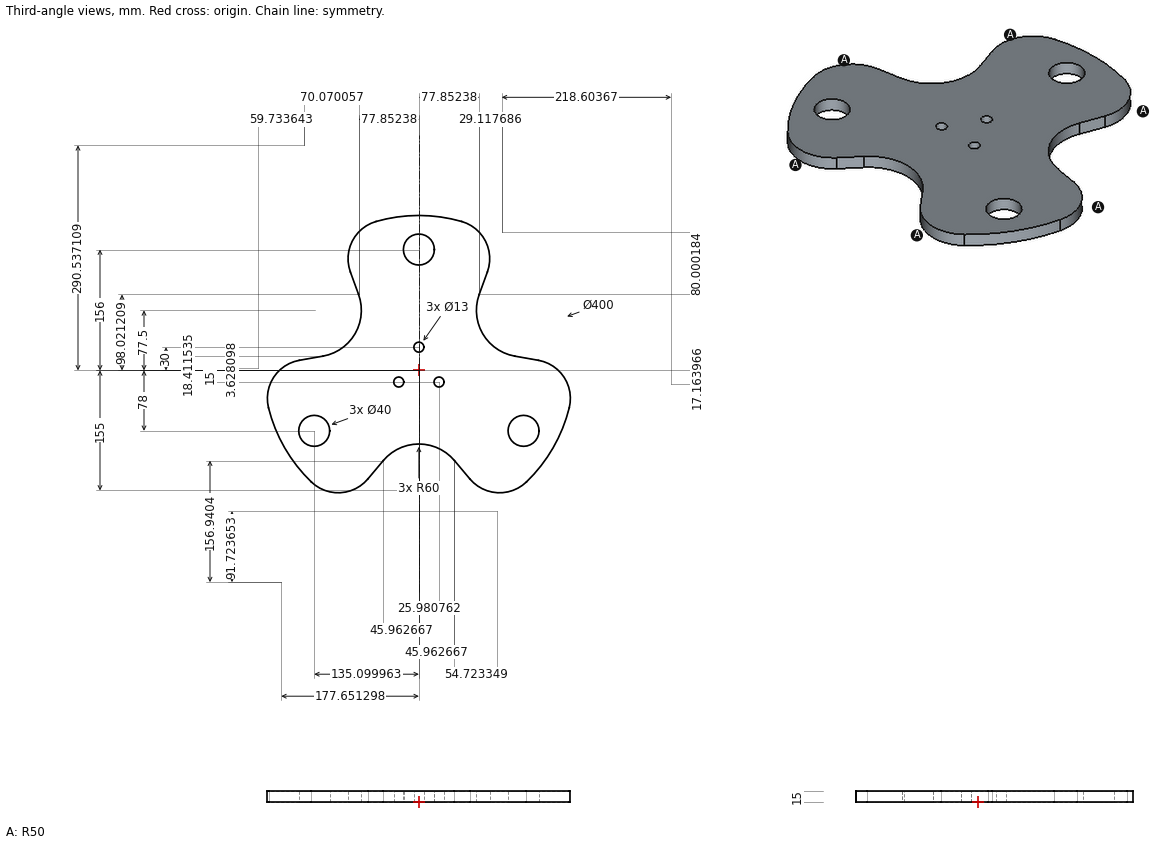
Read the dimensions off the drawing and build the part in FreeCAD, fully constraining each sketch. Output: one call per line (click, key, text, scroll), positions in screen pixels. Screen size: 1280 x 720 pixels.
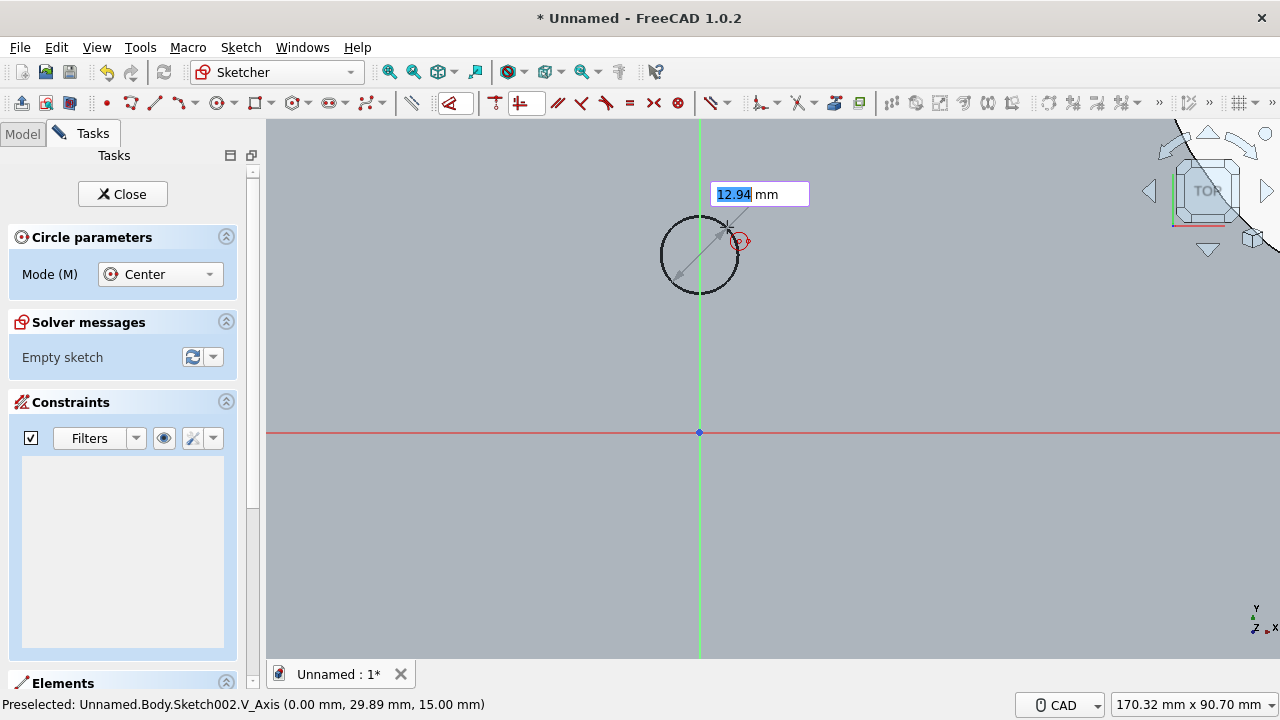
text(13)
key(Return)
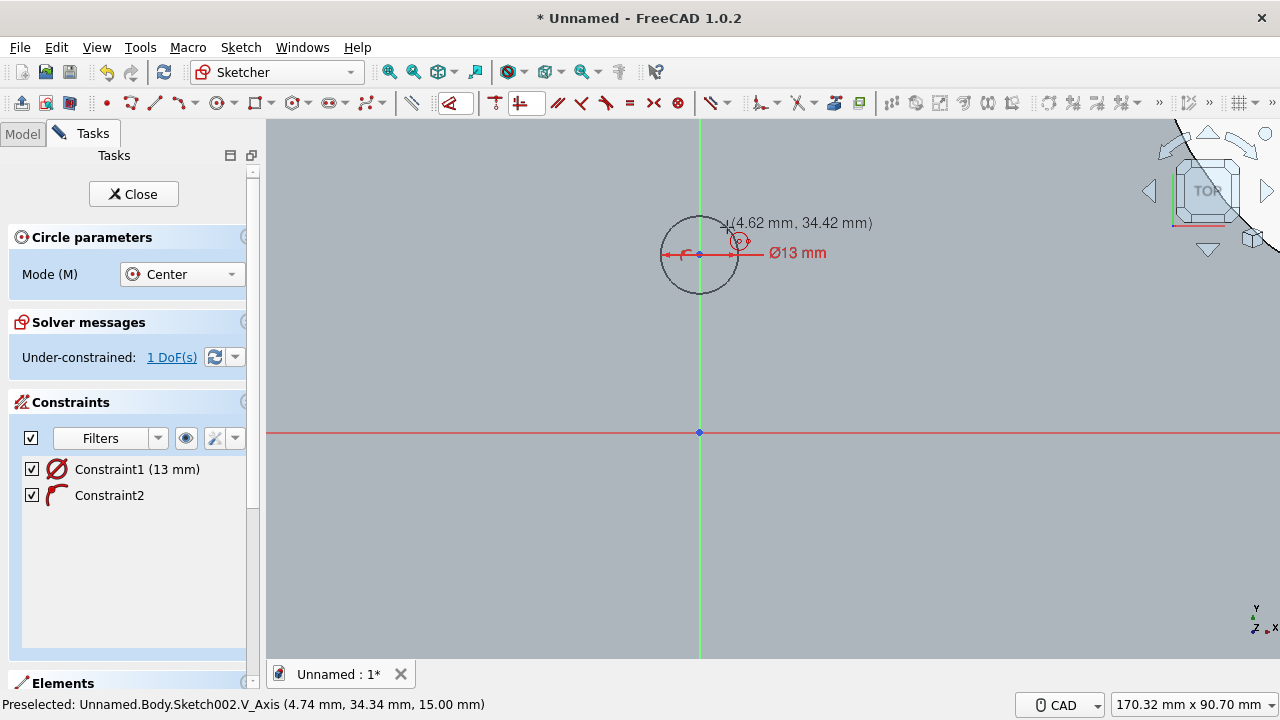
click(854, 522)
move(882, 495)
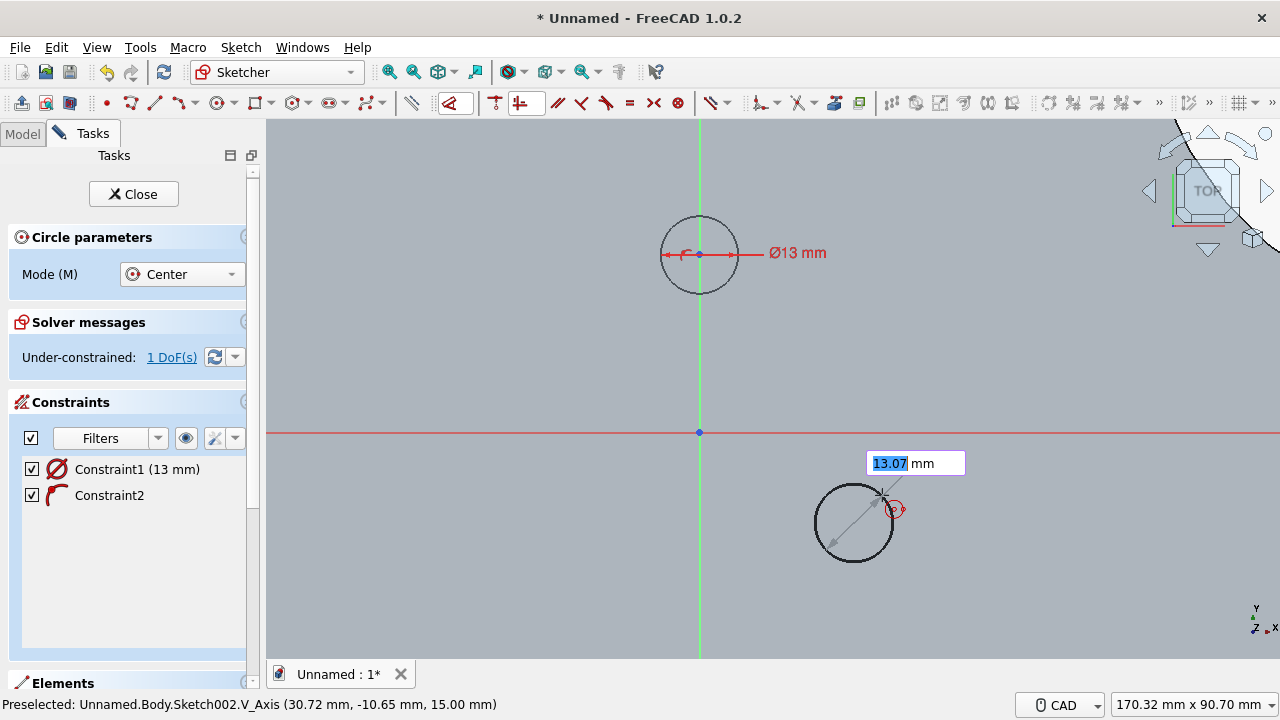
text(13)
key(Return)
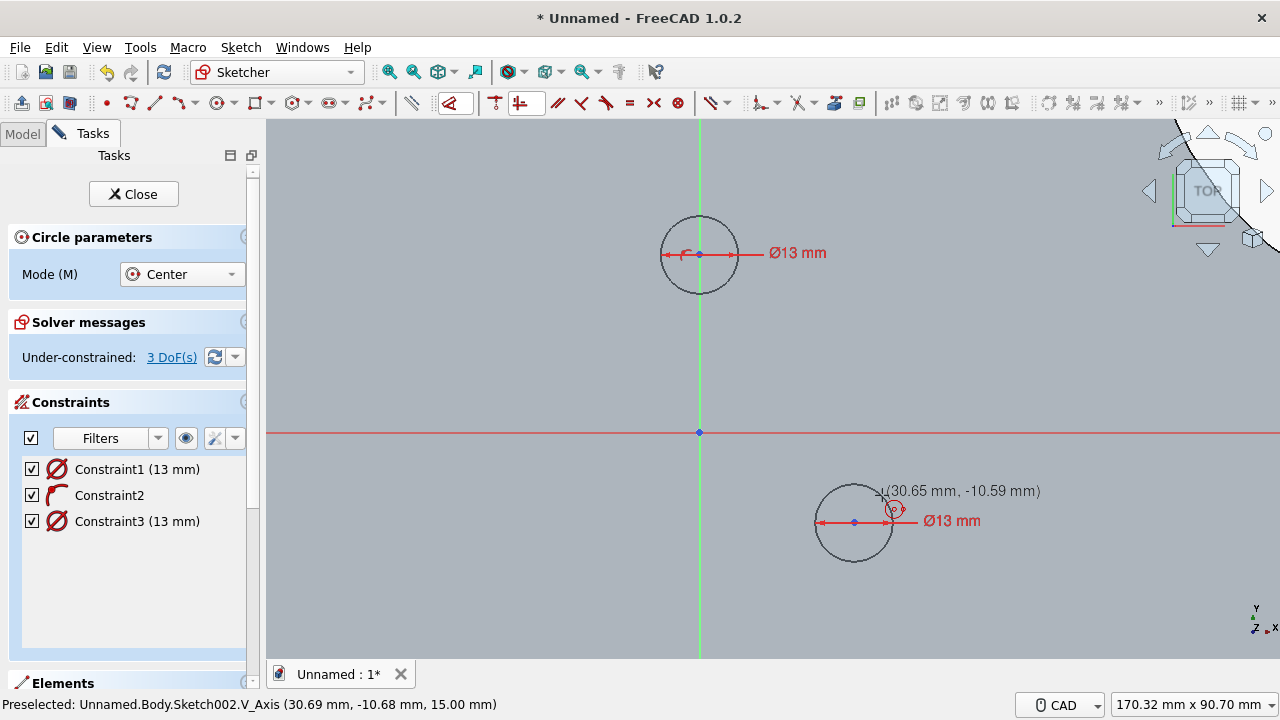
click(545, 522)
move(572, 495)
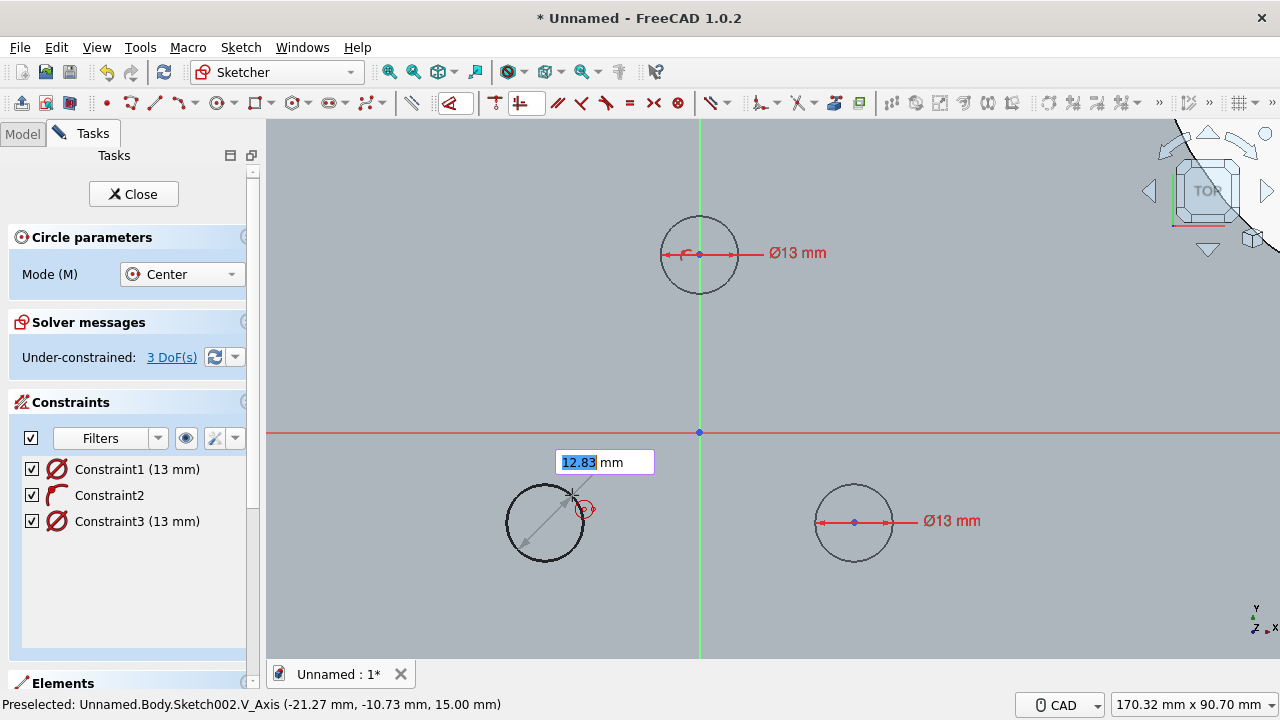
text(13)
key(Return)
key(Escape)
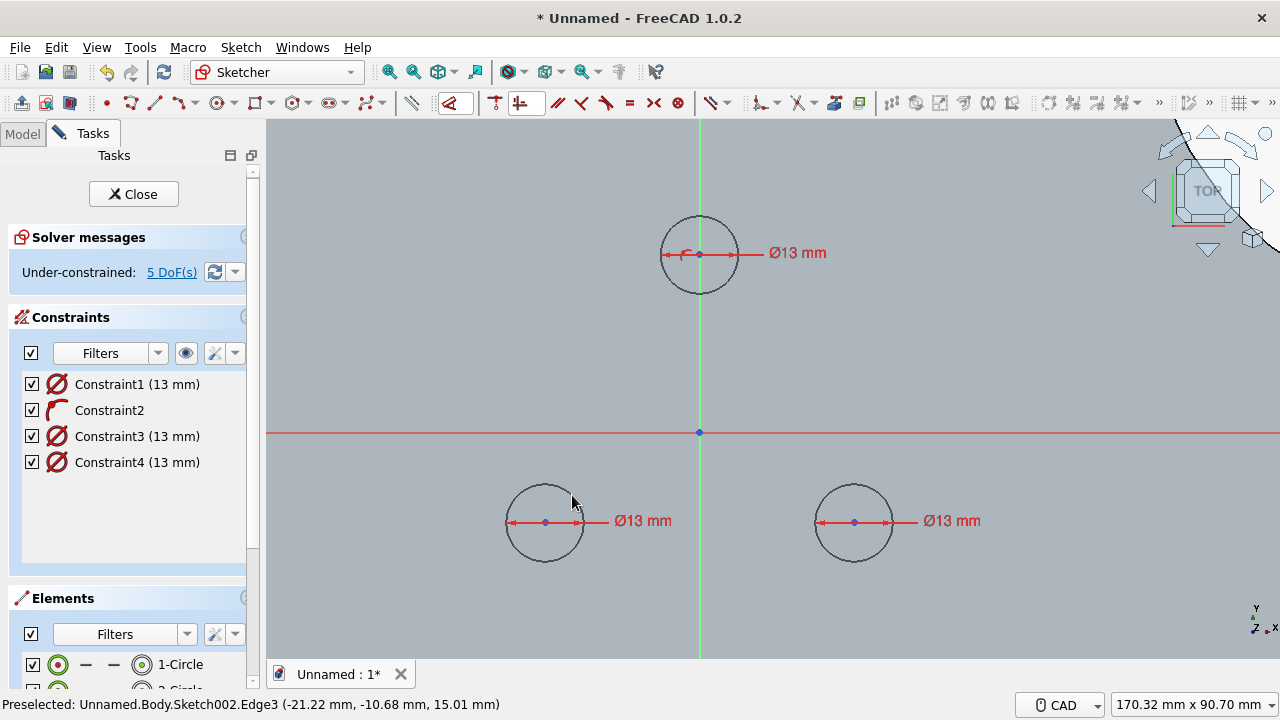
click(854, 523)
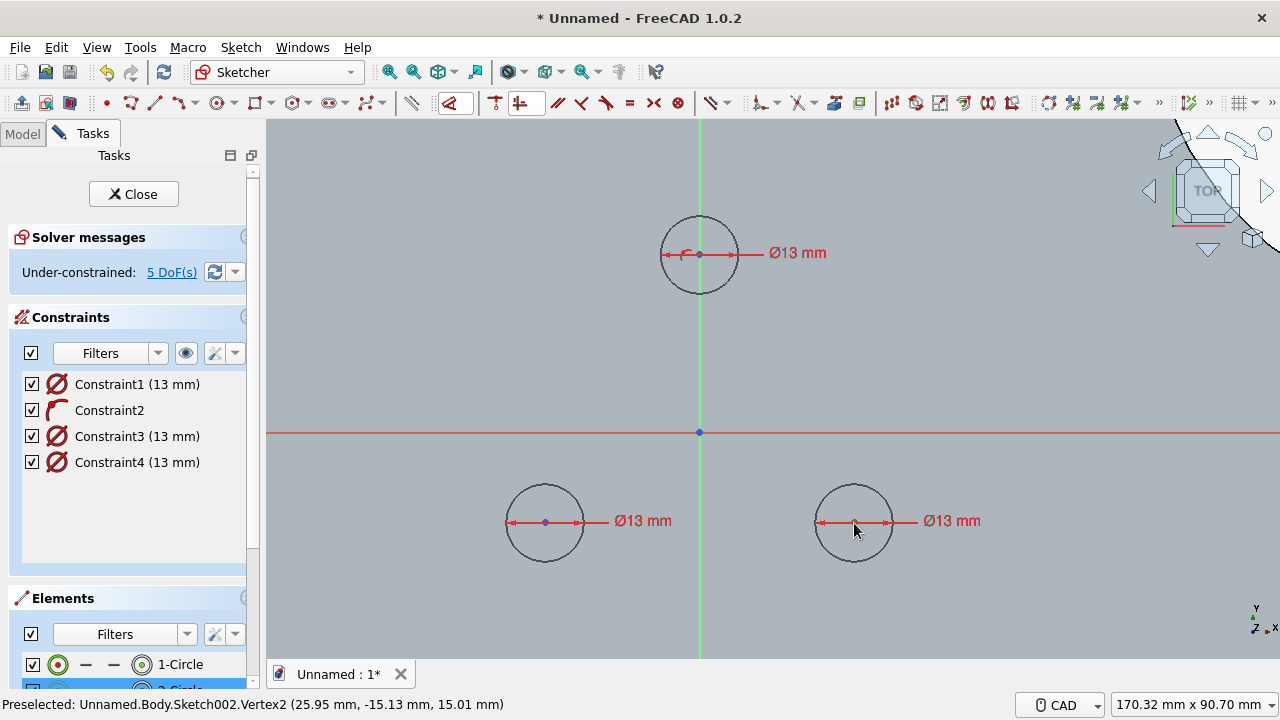
click(545, 523)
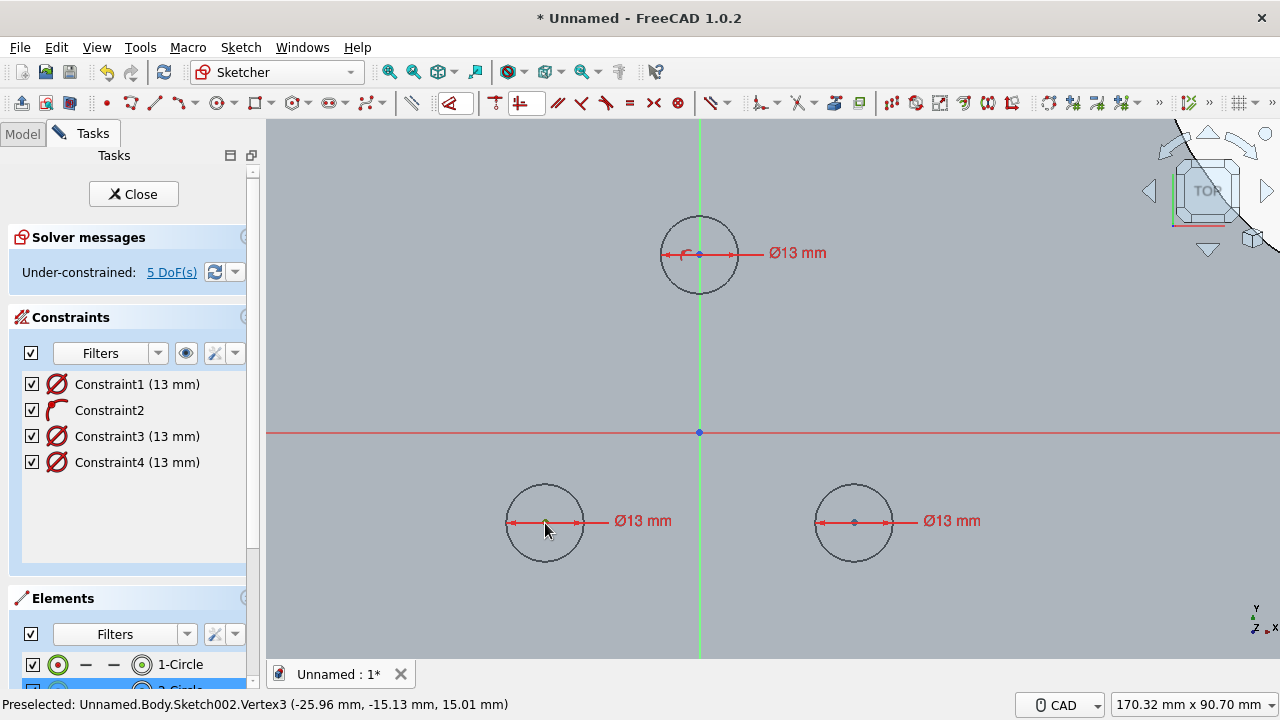
click(700, 596)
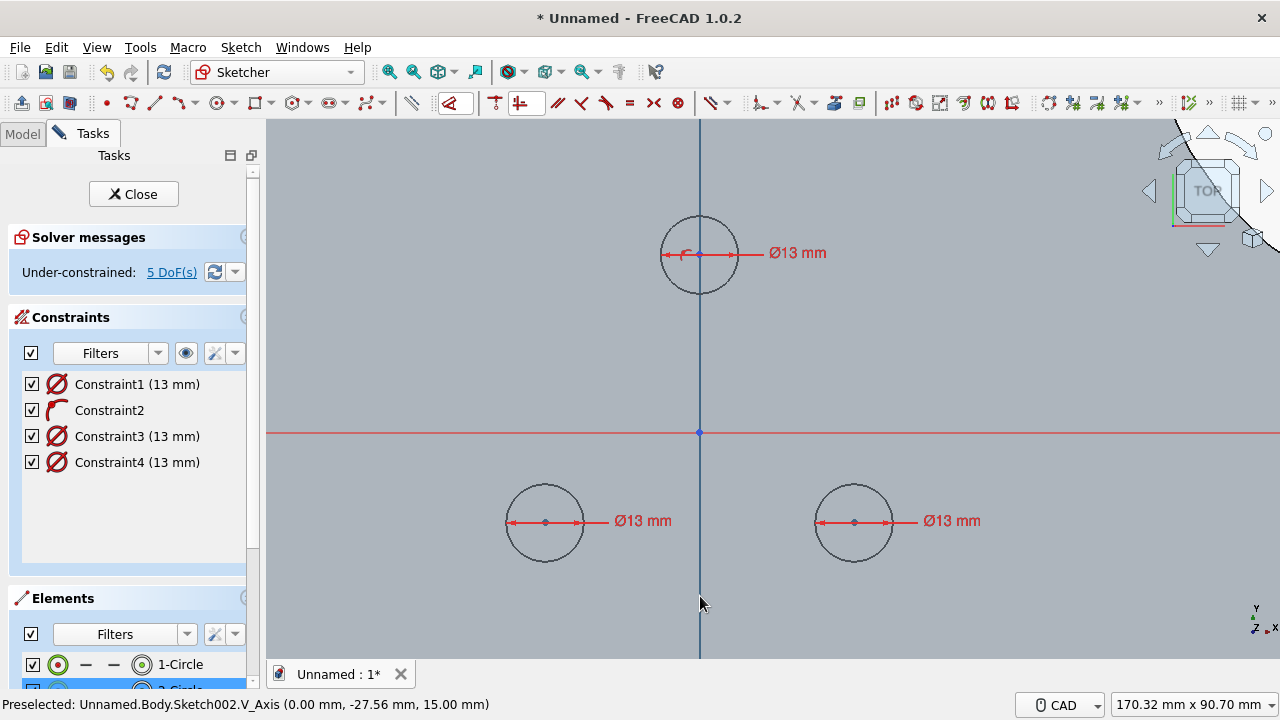
click(654, 104)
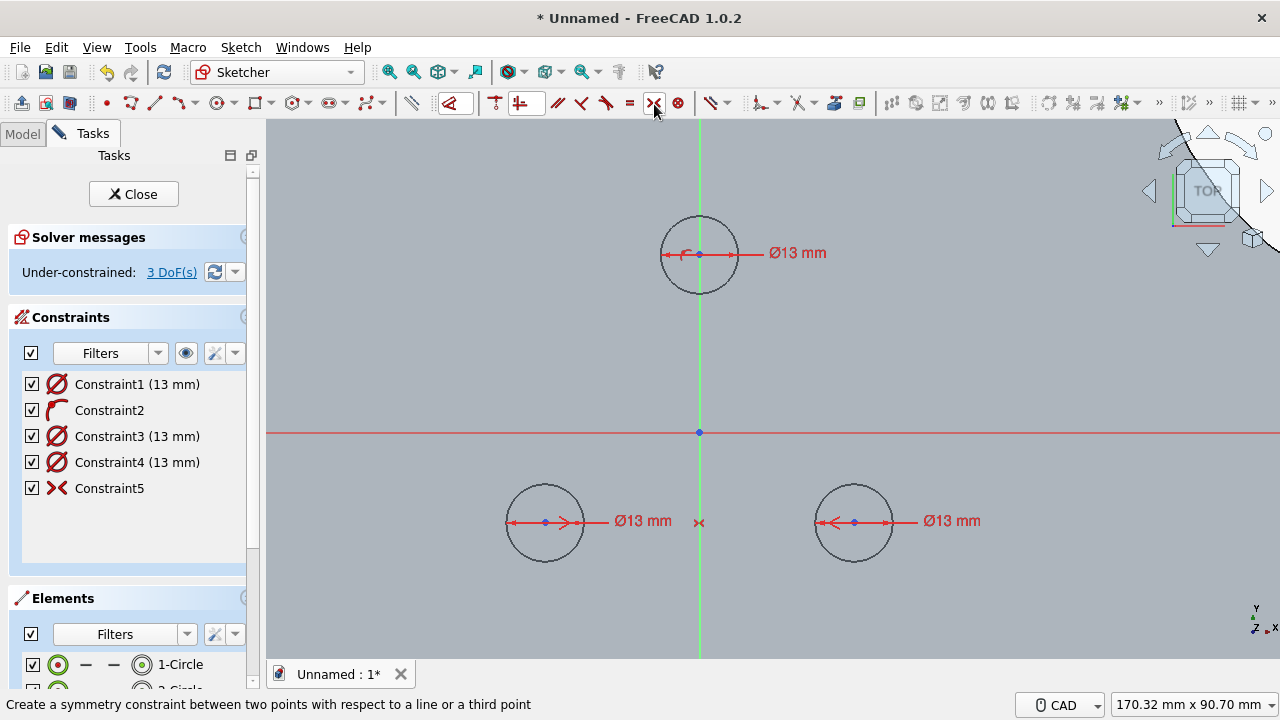
click(700, 255)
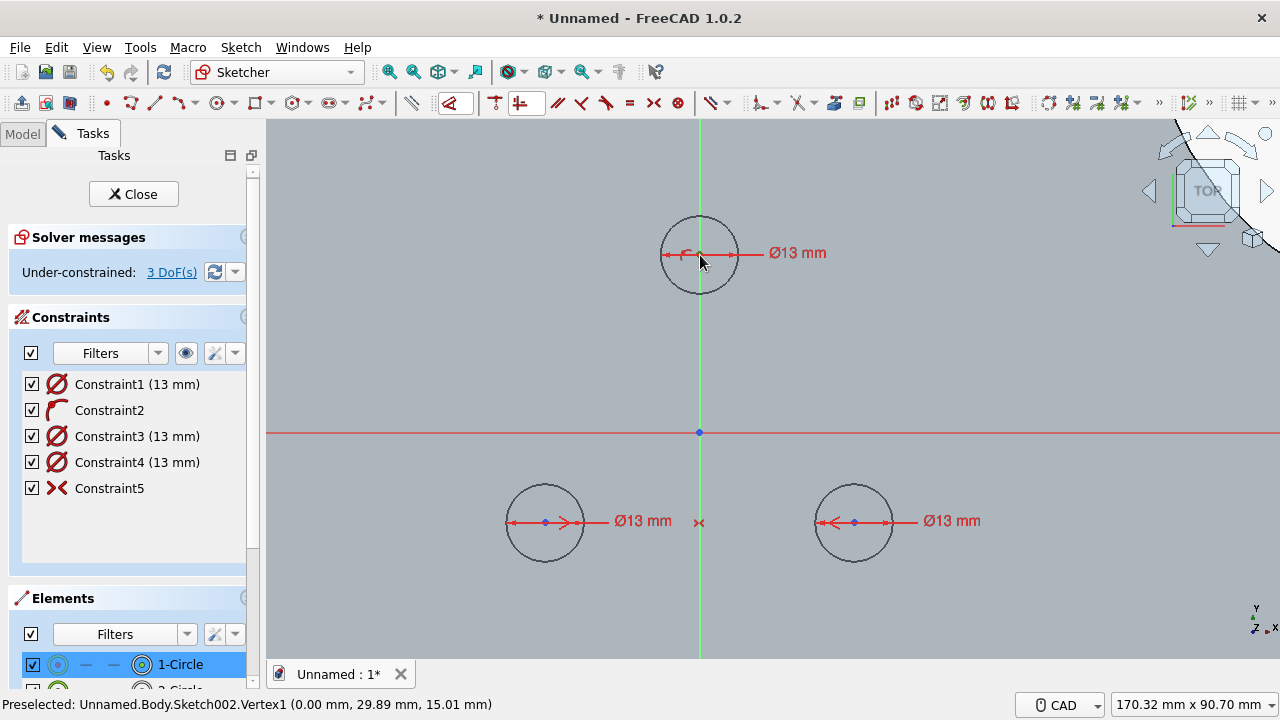
click(468, 104)